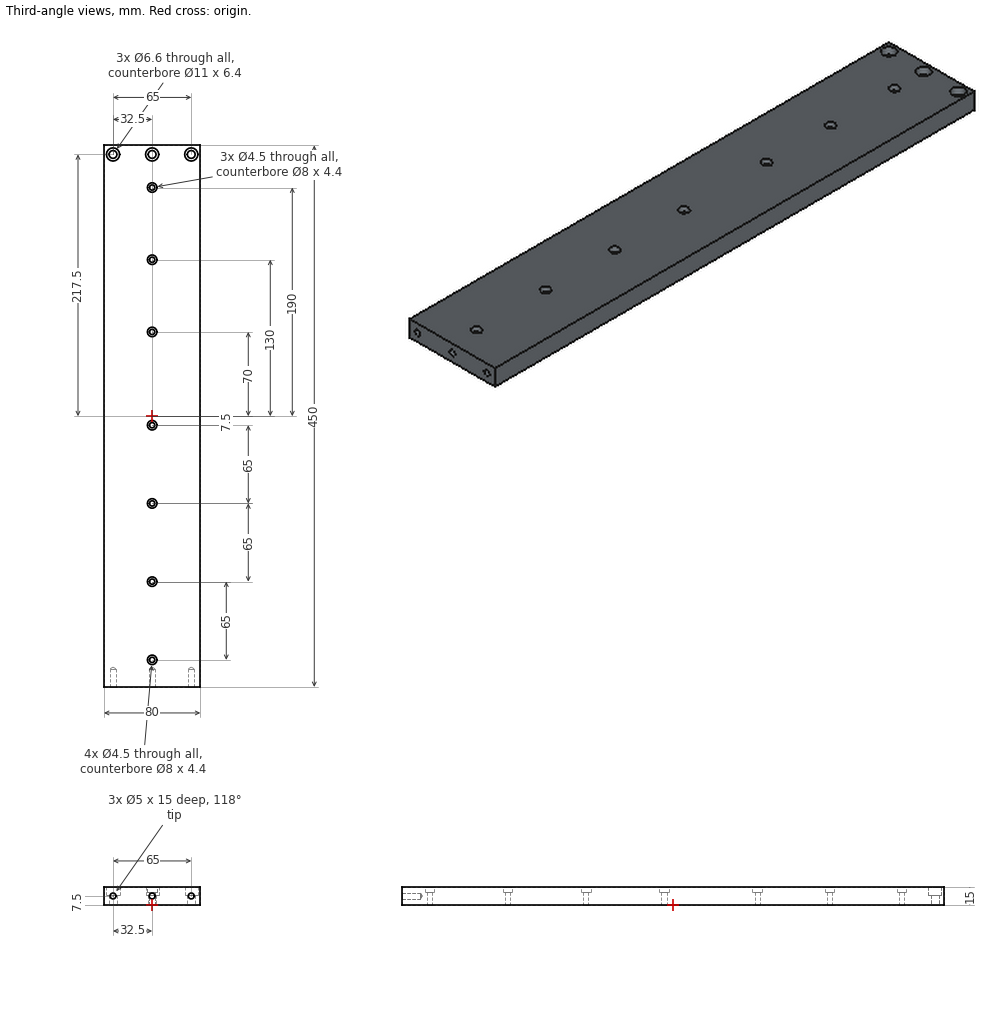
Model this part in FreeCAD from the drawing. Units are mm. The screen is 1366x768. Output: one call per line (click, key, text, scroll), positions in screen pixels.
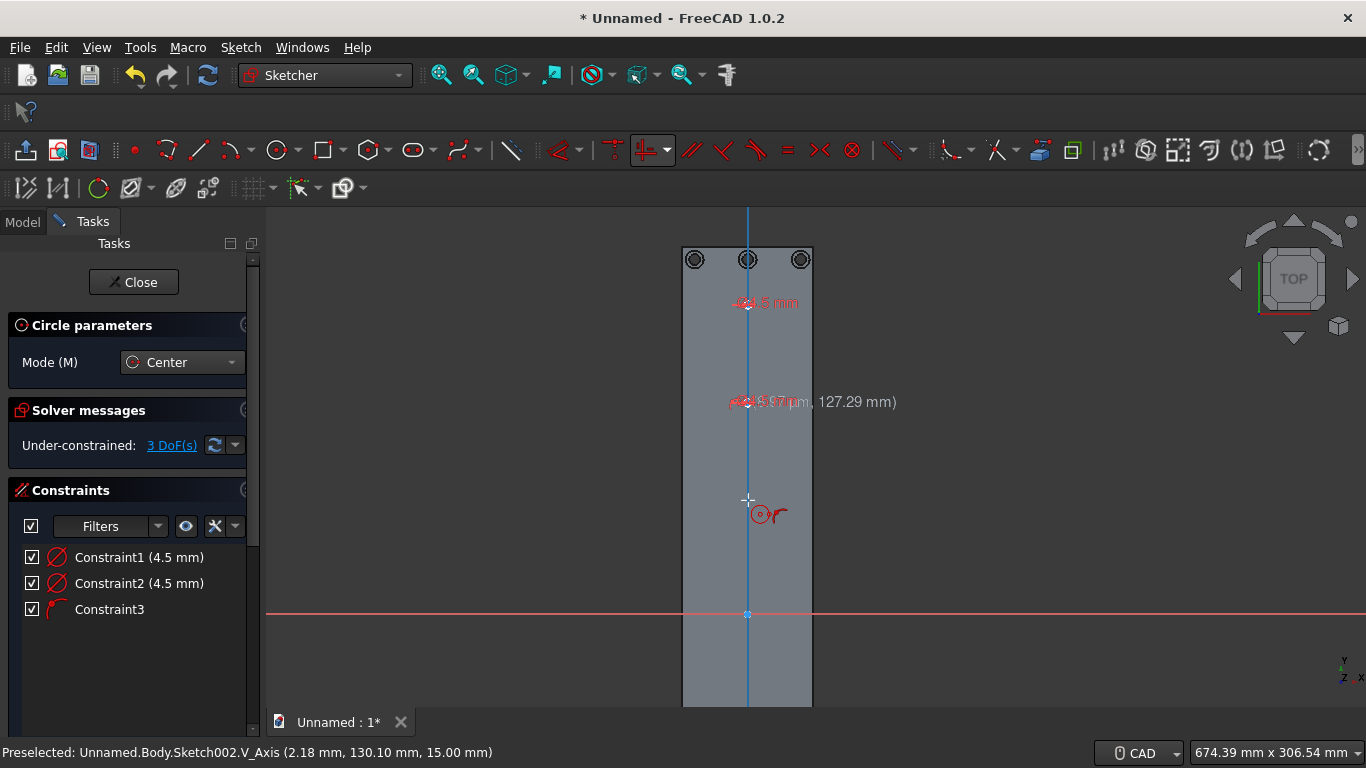
click(748, 500)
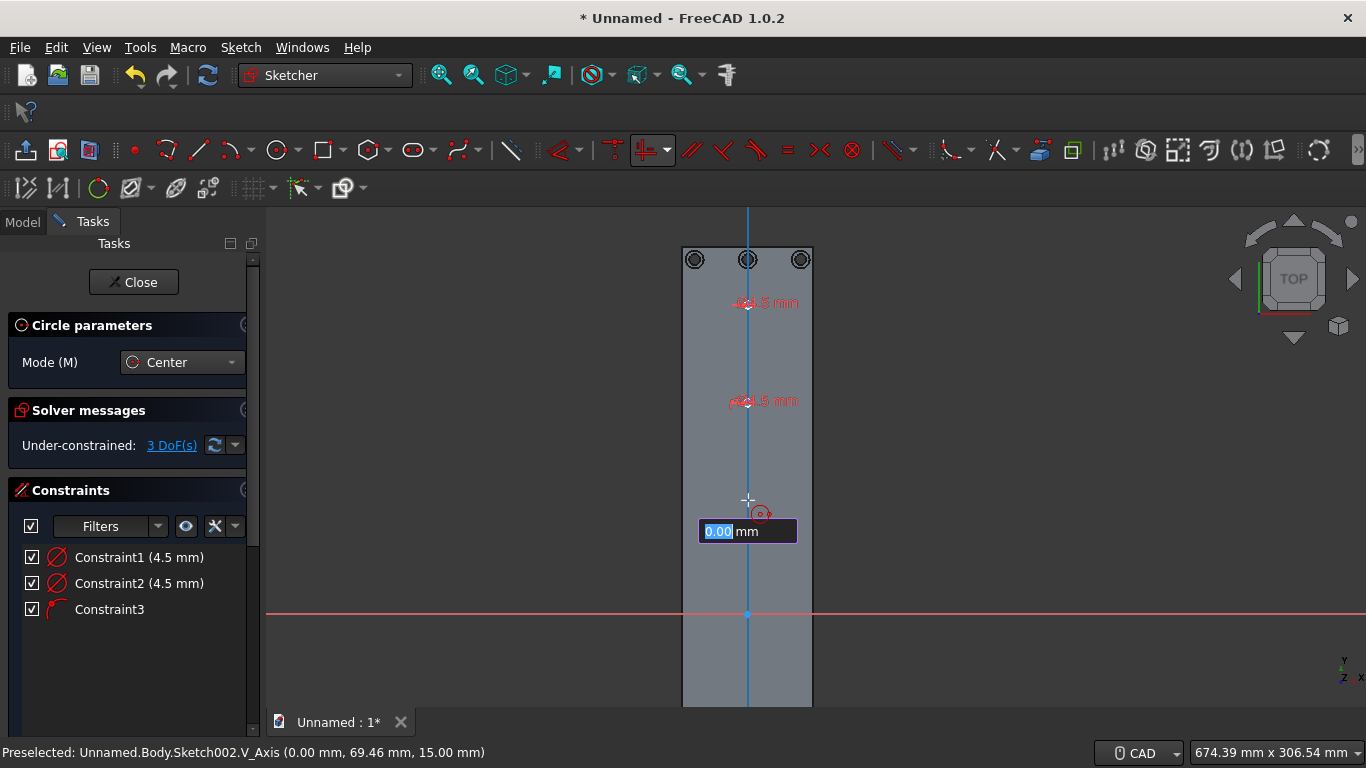
scroll(751, 499, up, 8)
move(750, 496)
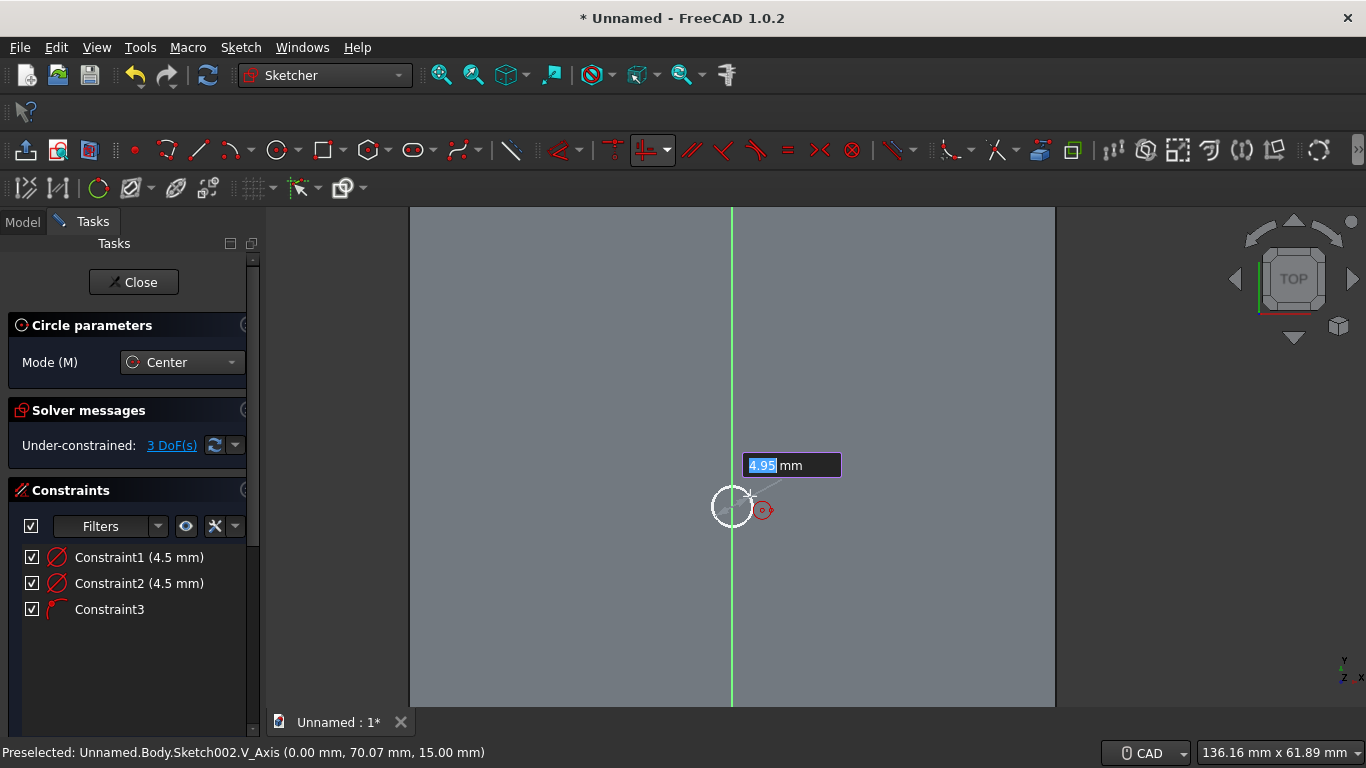
text(4.5)
key(Return)
key(Escape)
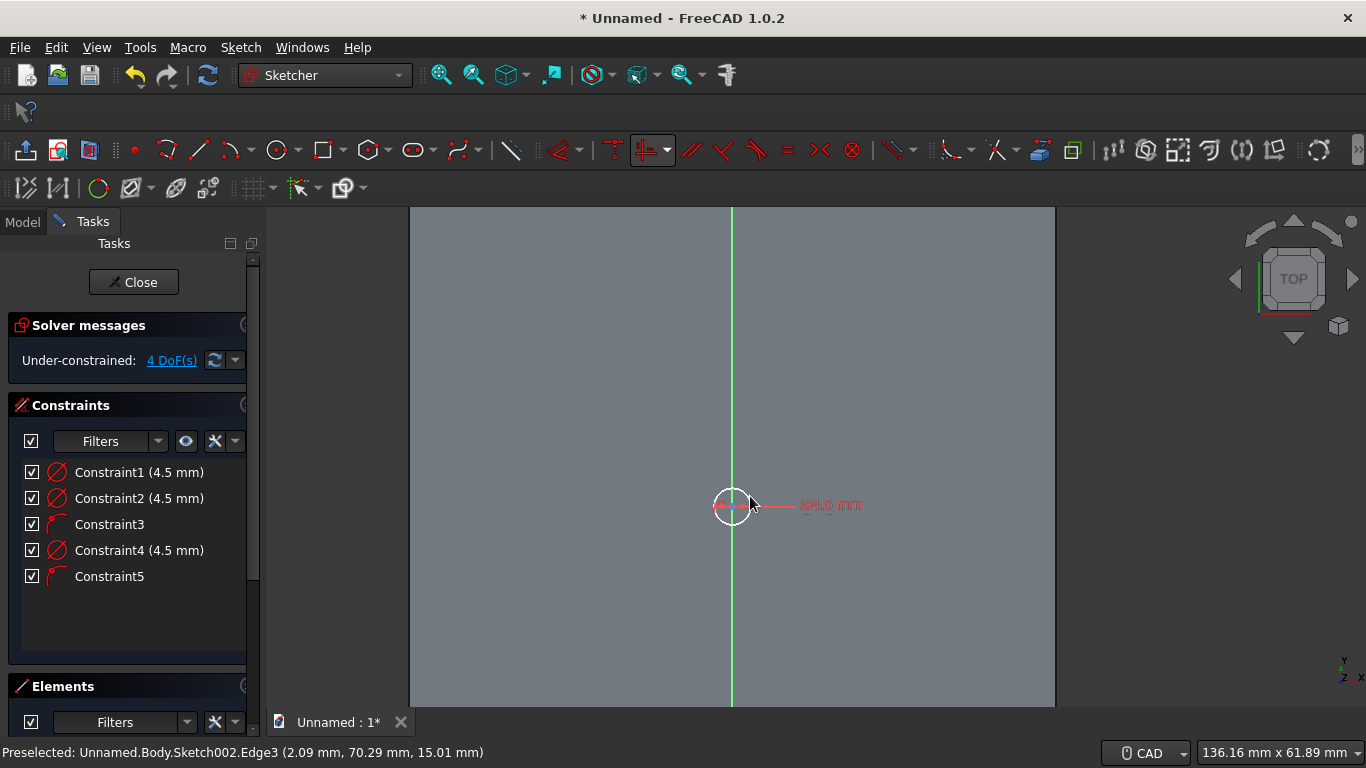
scroll(751, 499, down, 8)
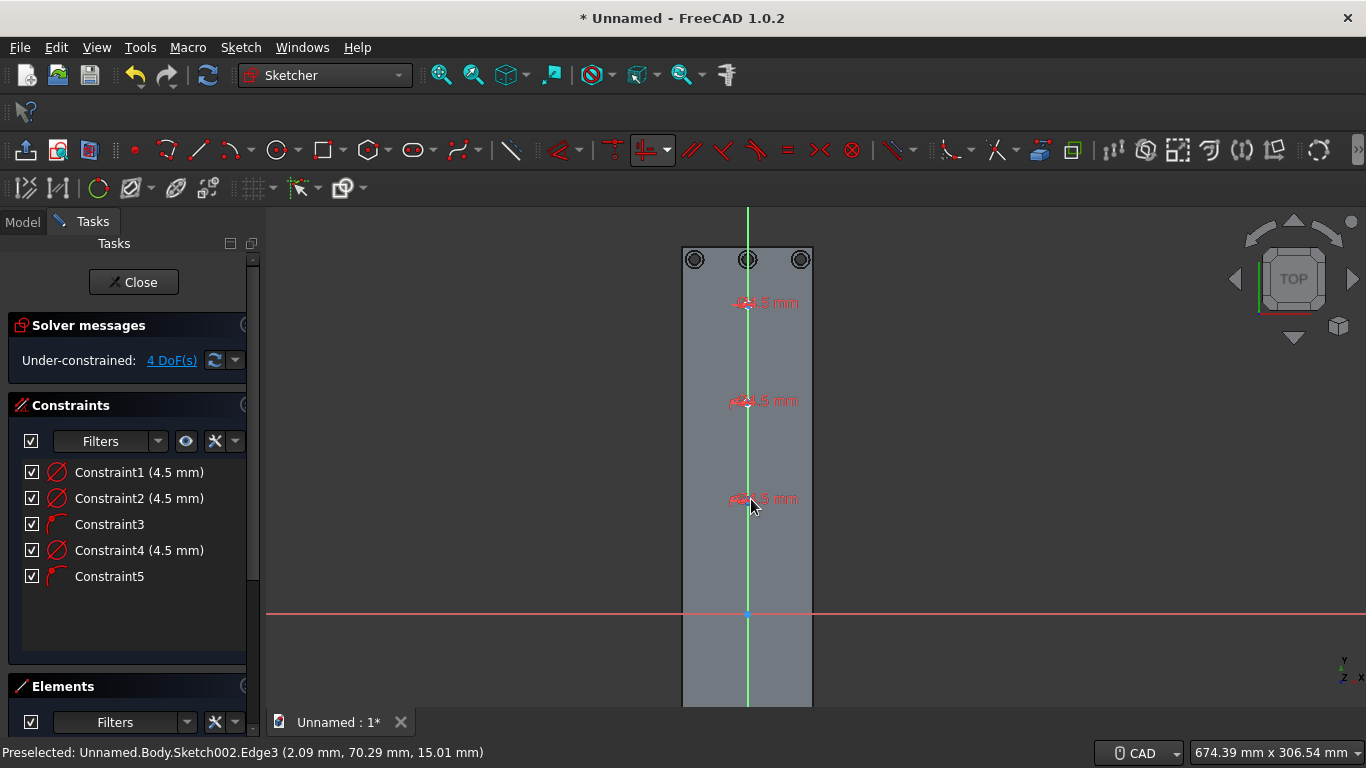
click(748, 305)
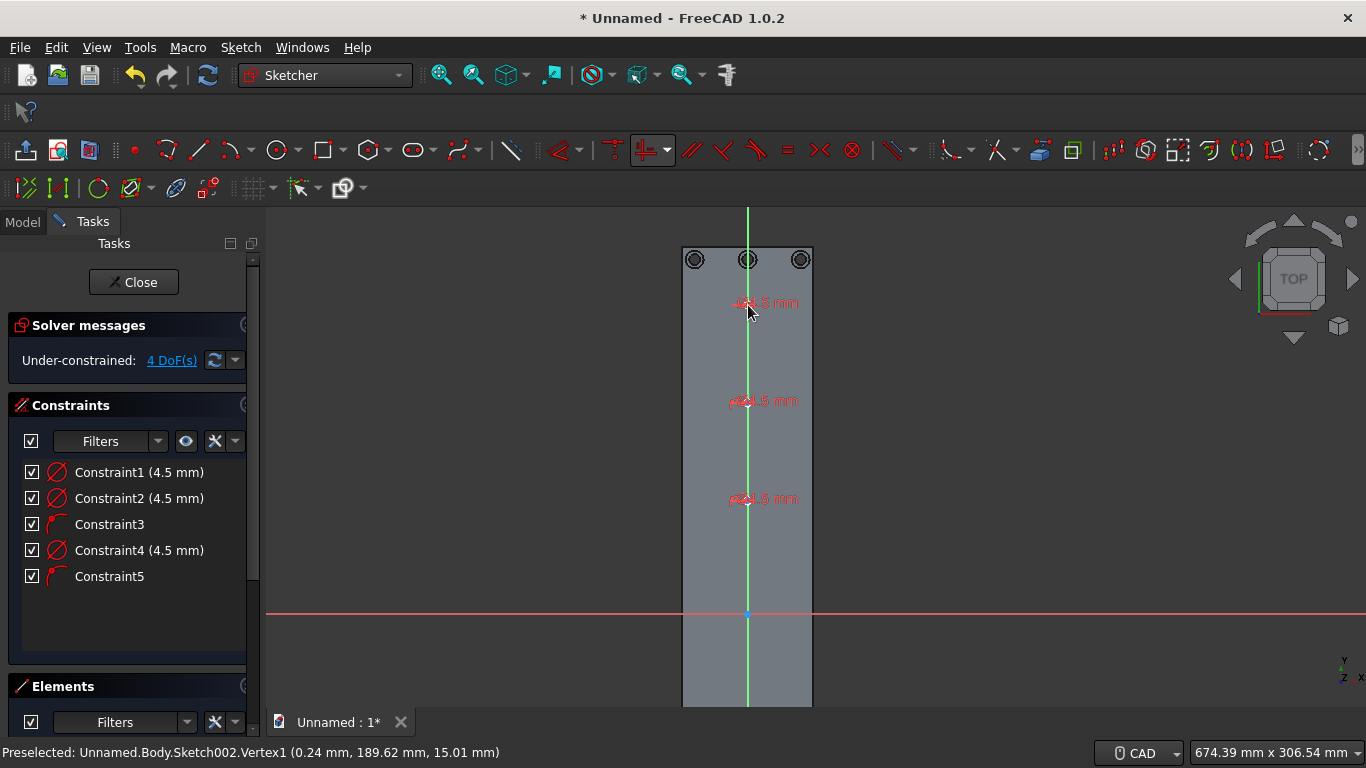
click(748, 647)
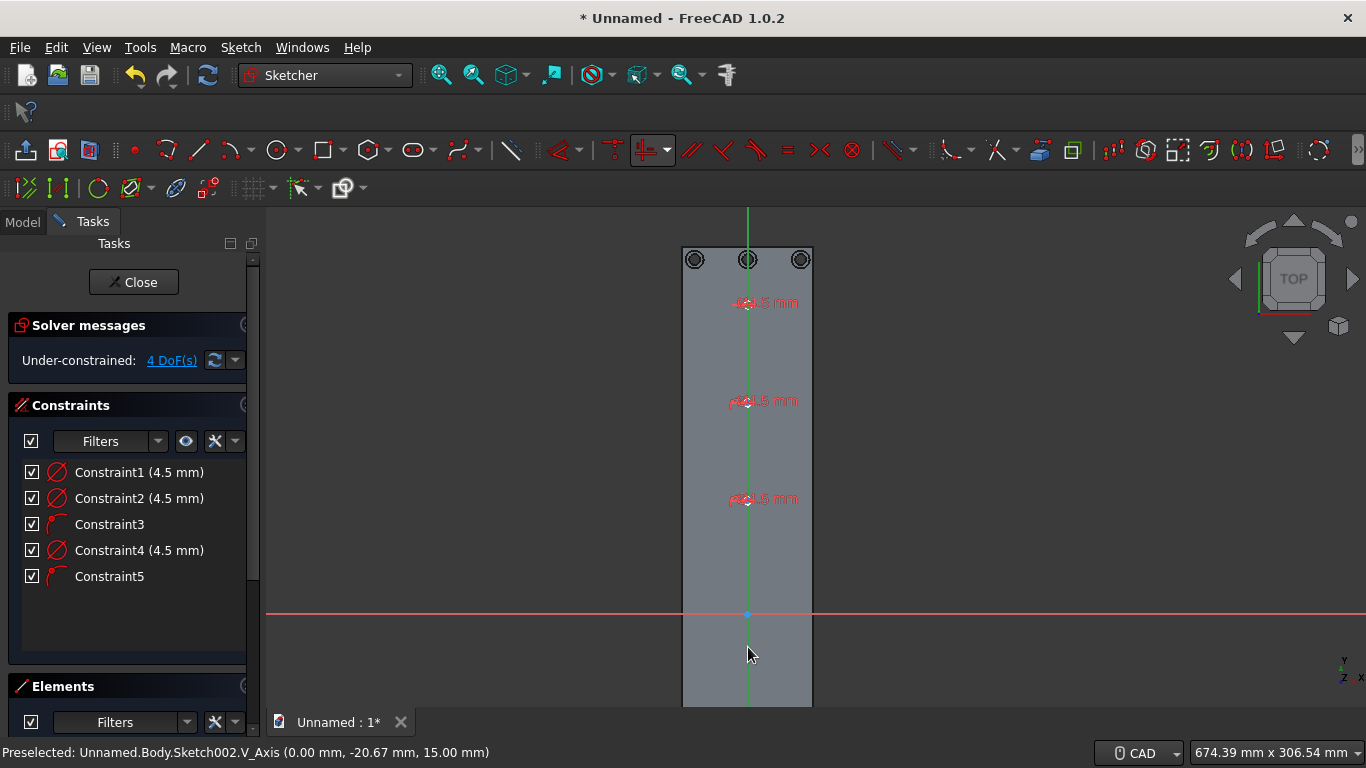
click(614, 150)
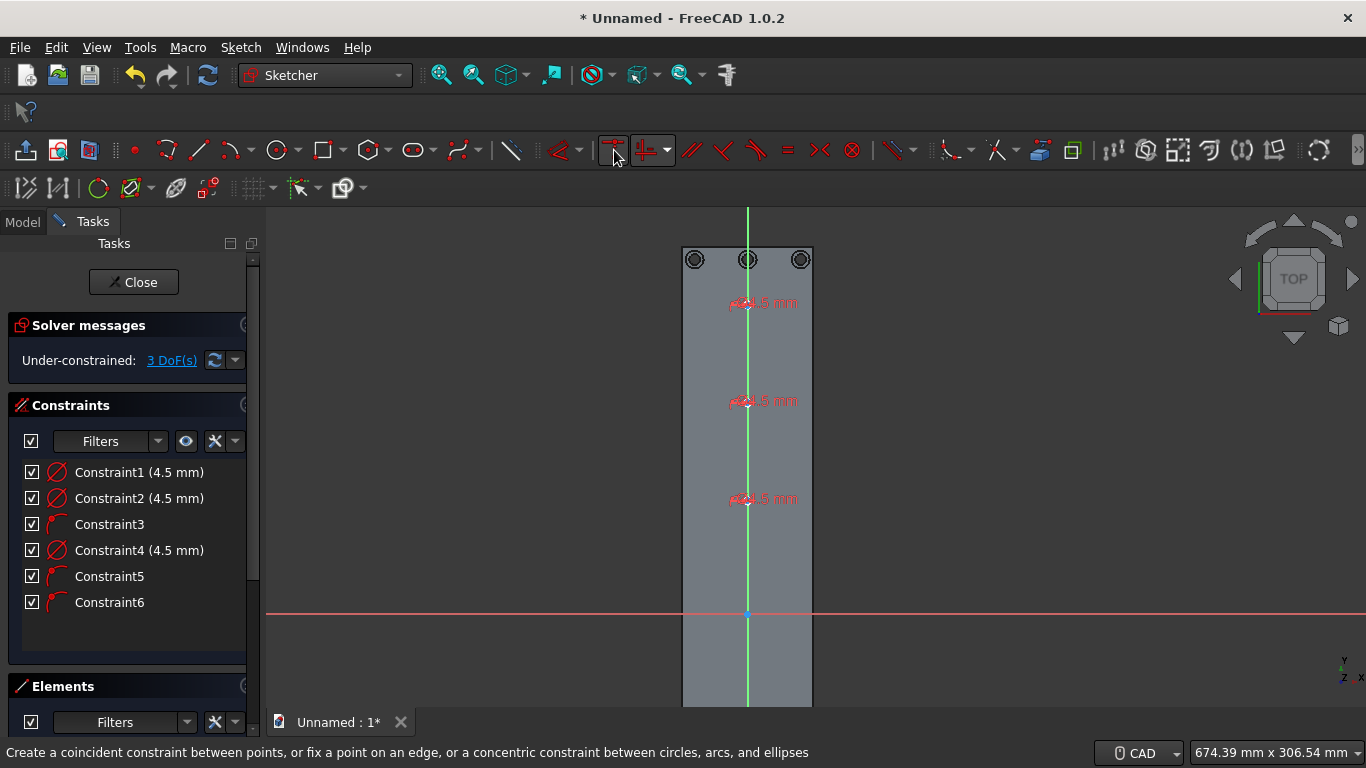
click(558, 150)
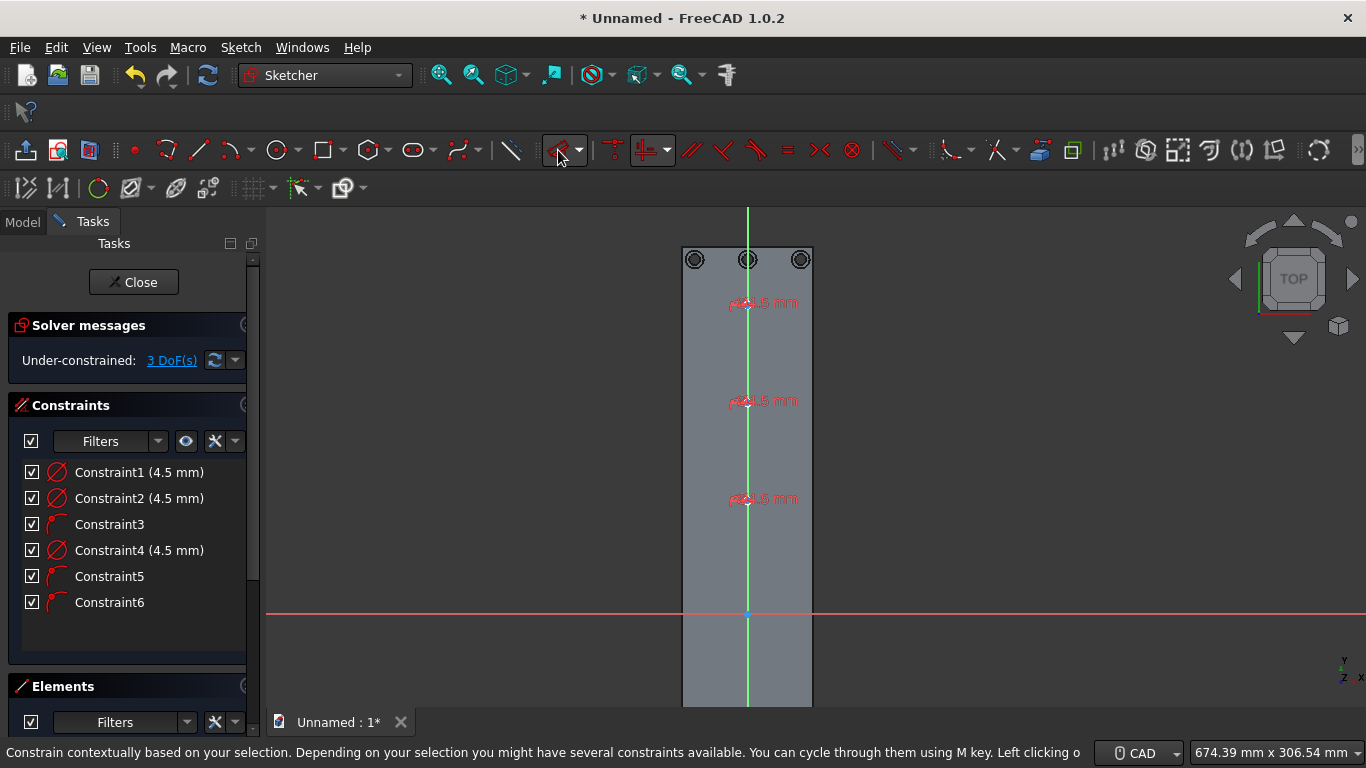
click(748, 501)
click(782, 558)